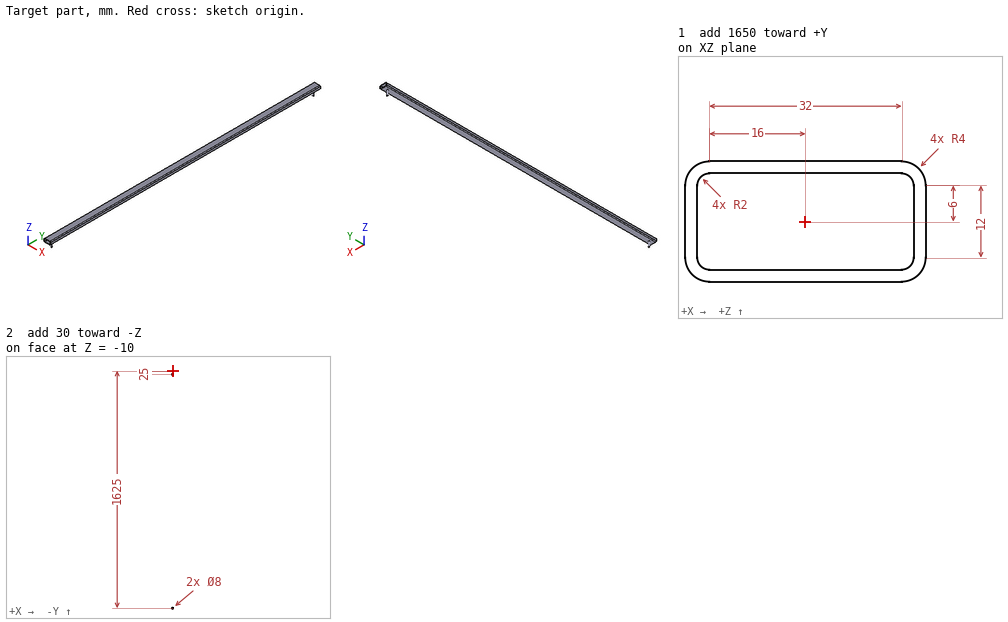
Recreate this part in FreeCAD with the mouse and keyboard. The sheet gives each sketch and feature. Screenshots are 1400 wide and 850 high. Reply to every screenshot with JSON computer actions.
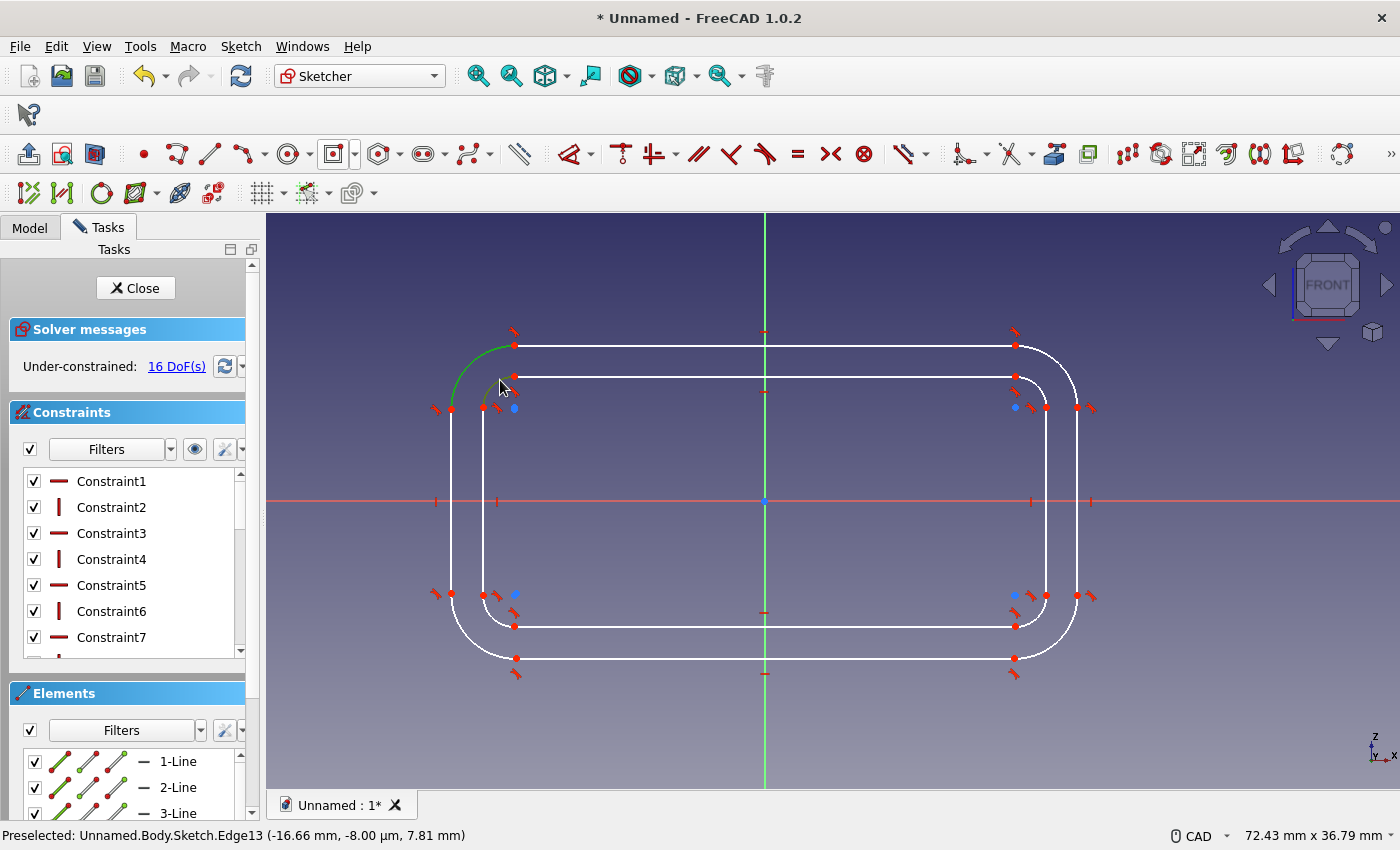
{"action": "left_click", "coordinate": [621, 154]}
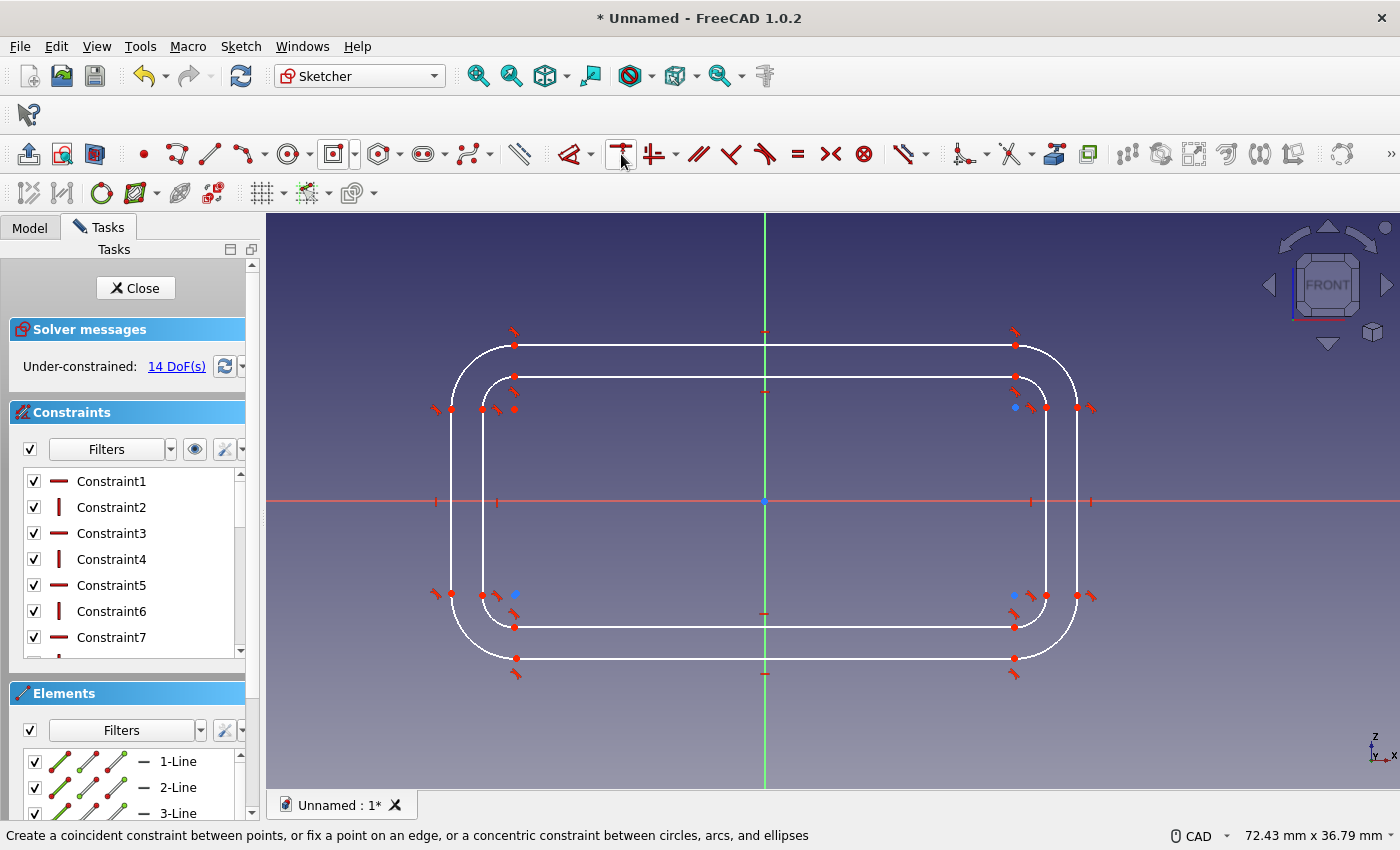
{"action": "left_click", "coordinate": [458, 623]}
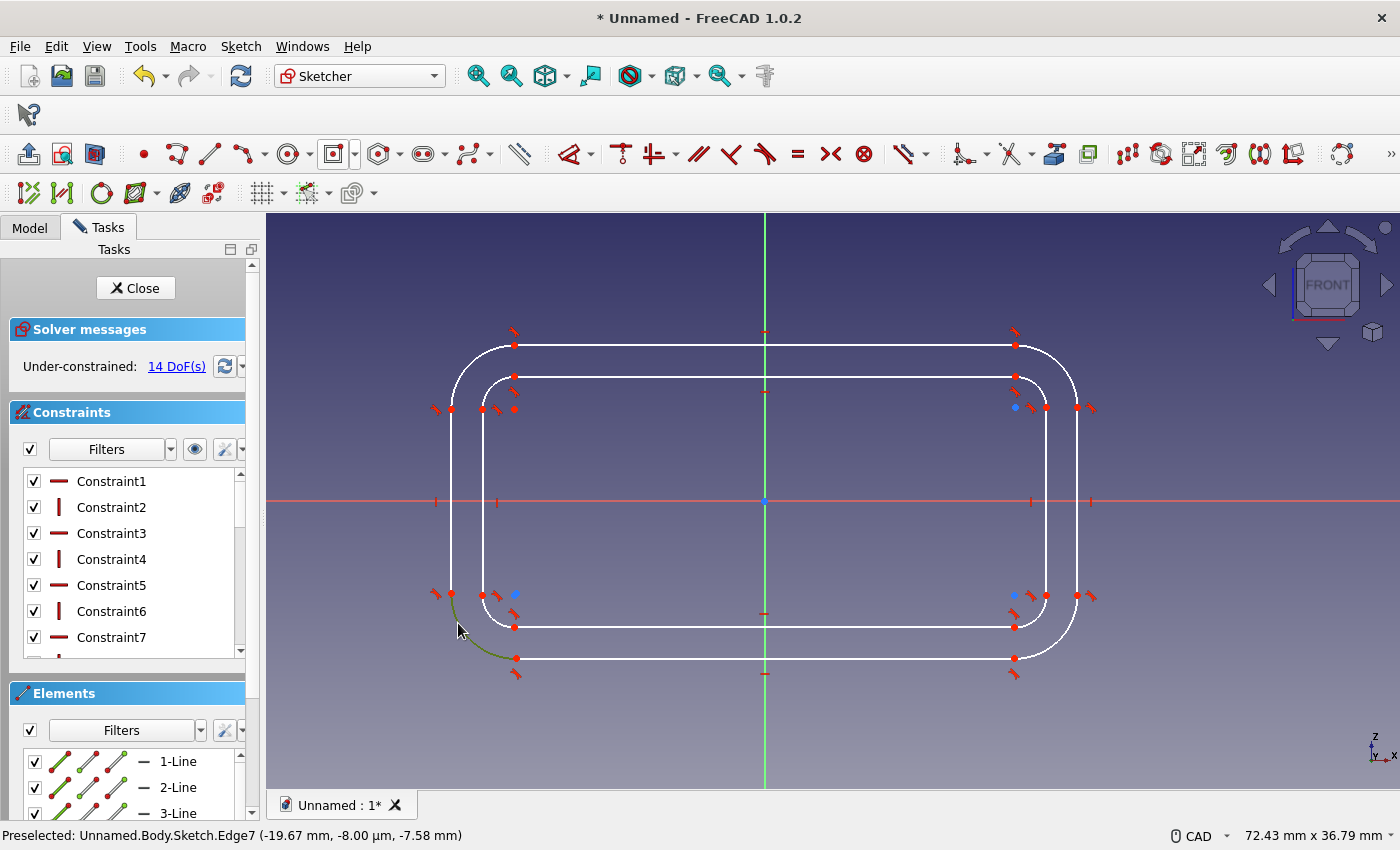
{"action": "left_click", "coordinate": [486, 610]}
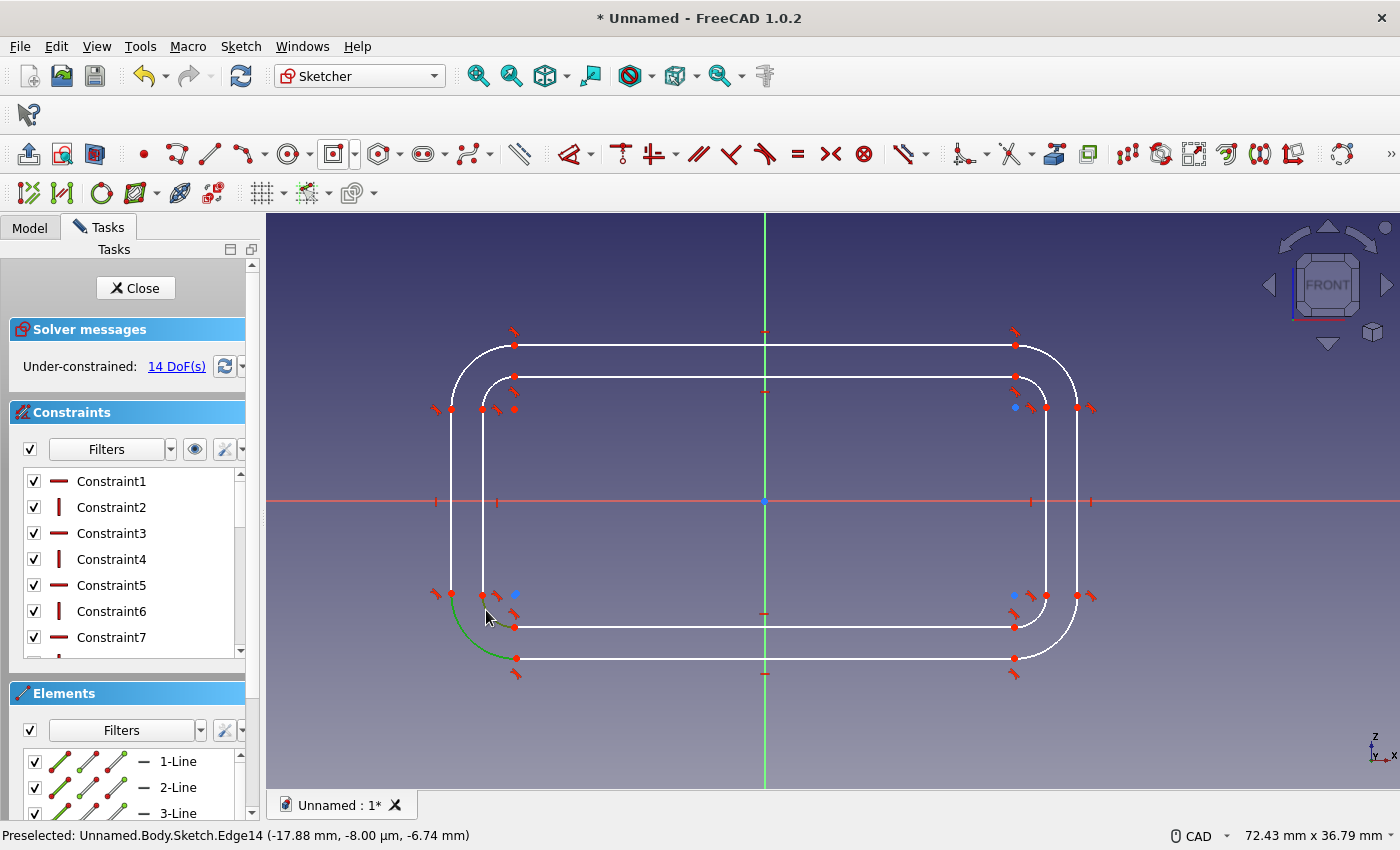
{"action": "key", "text": "c"}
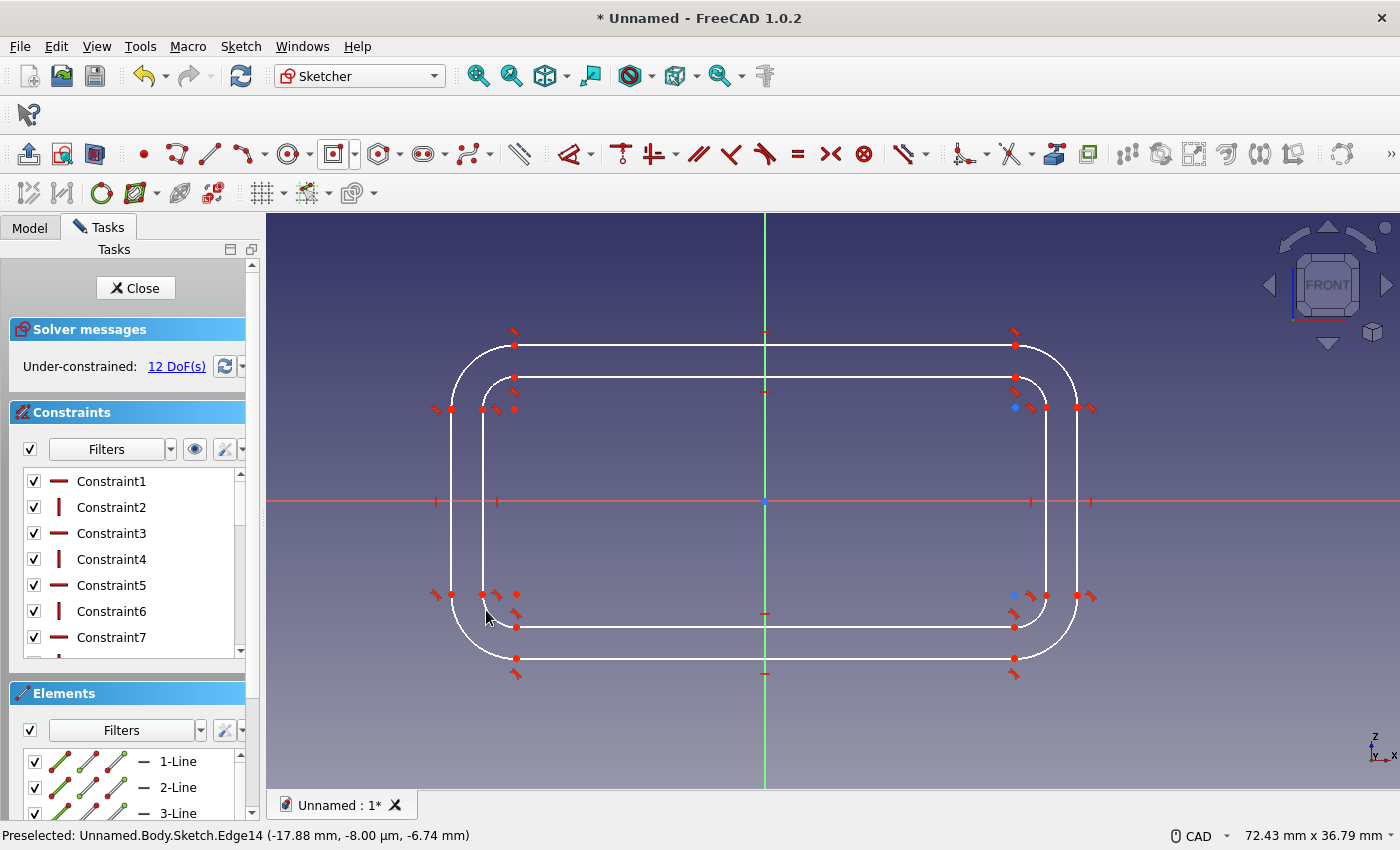
{"action": "left_click", "coordinate": [1043, 652]}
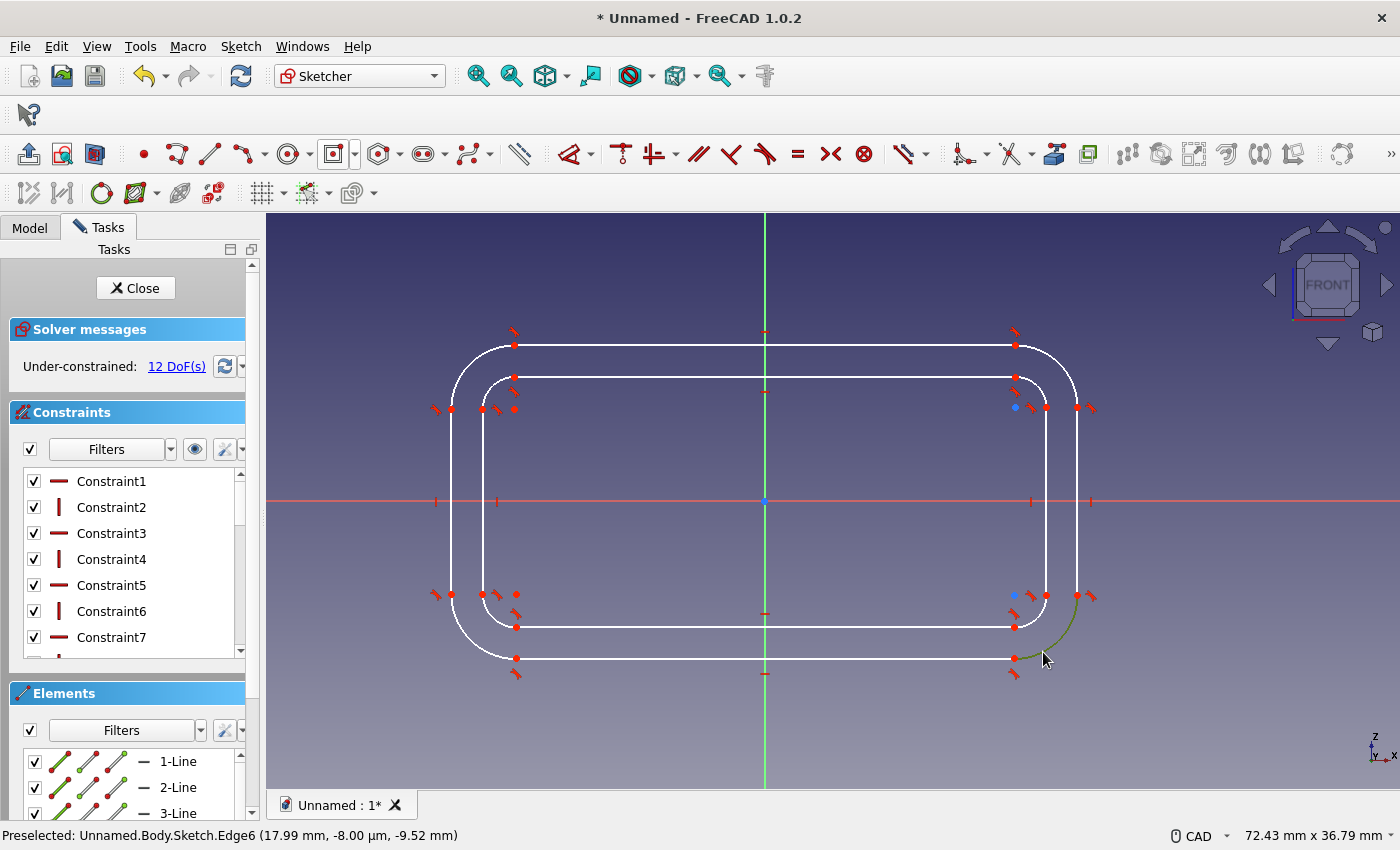
{"action": "left_click", "coordinate": [1029, 624]}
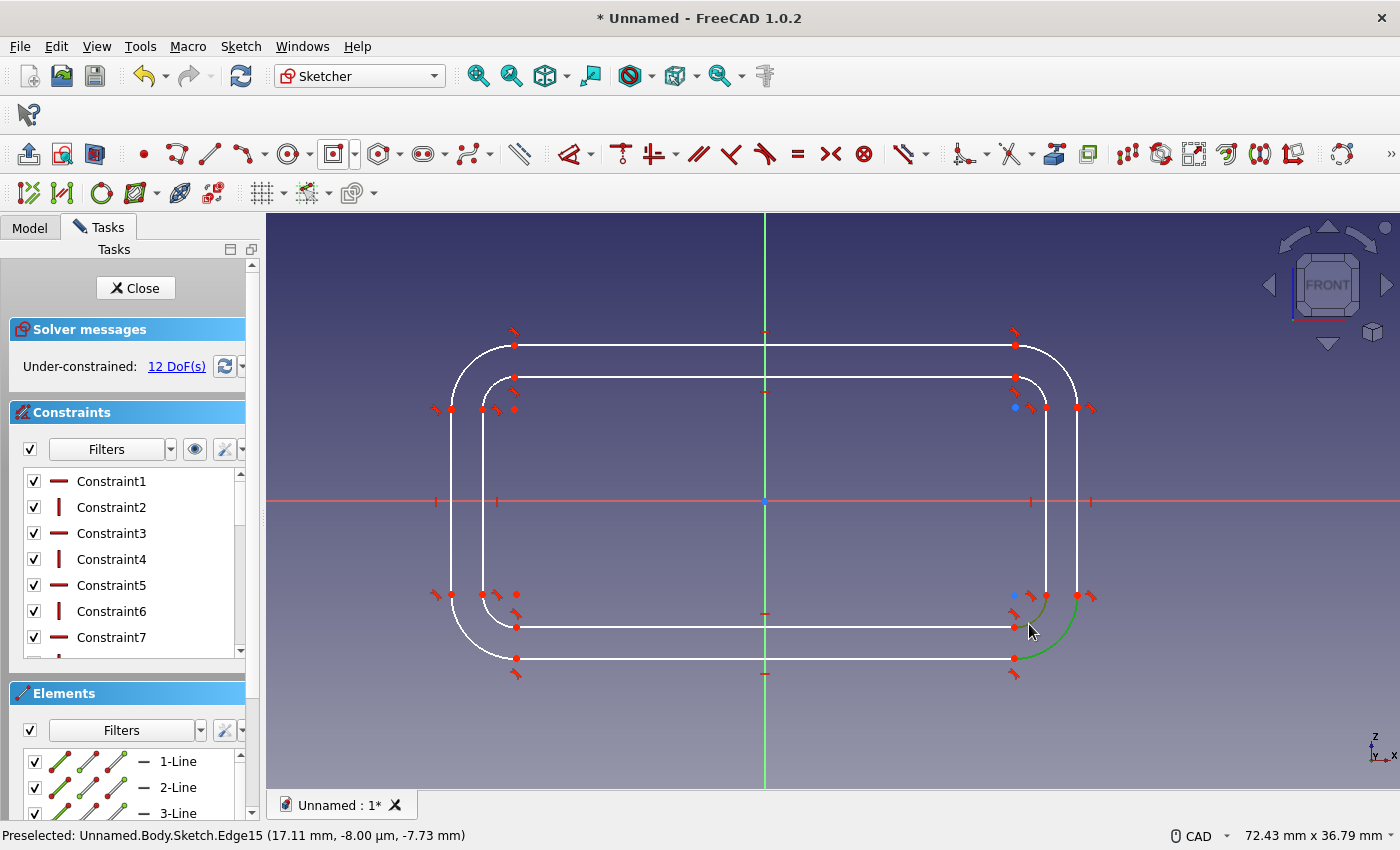
{"action": "left_click", "coordinate": [621, 154]}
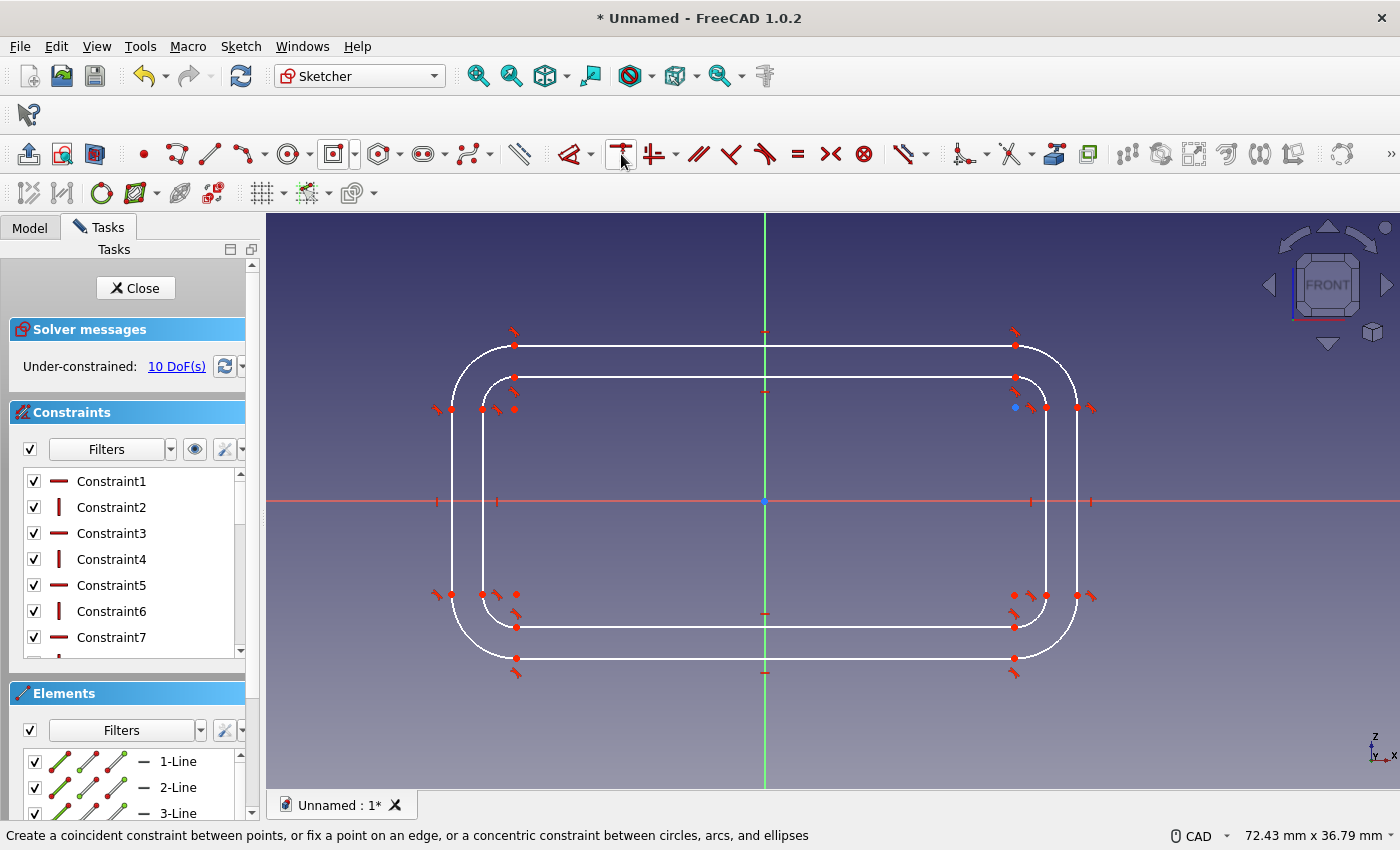
{"action": "left_click", "coordinate": [1071, 380]}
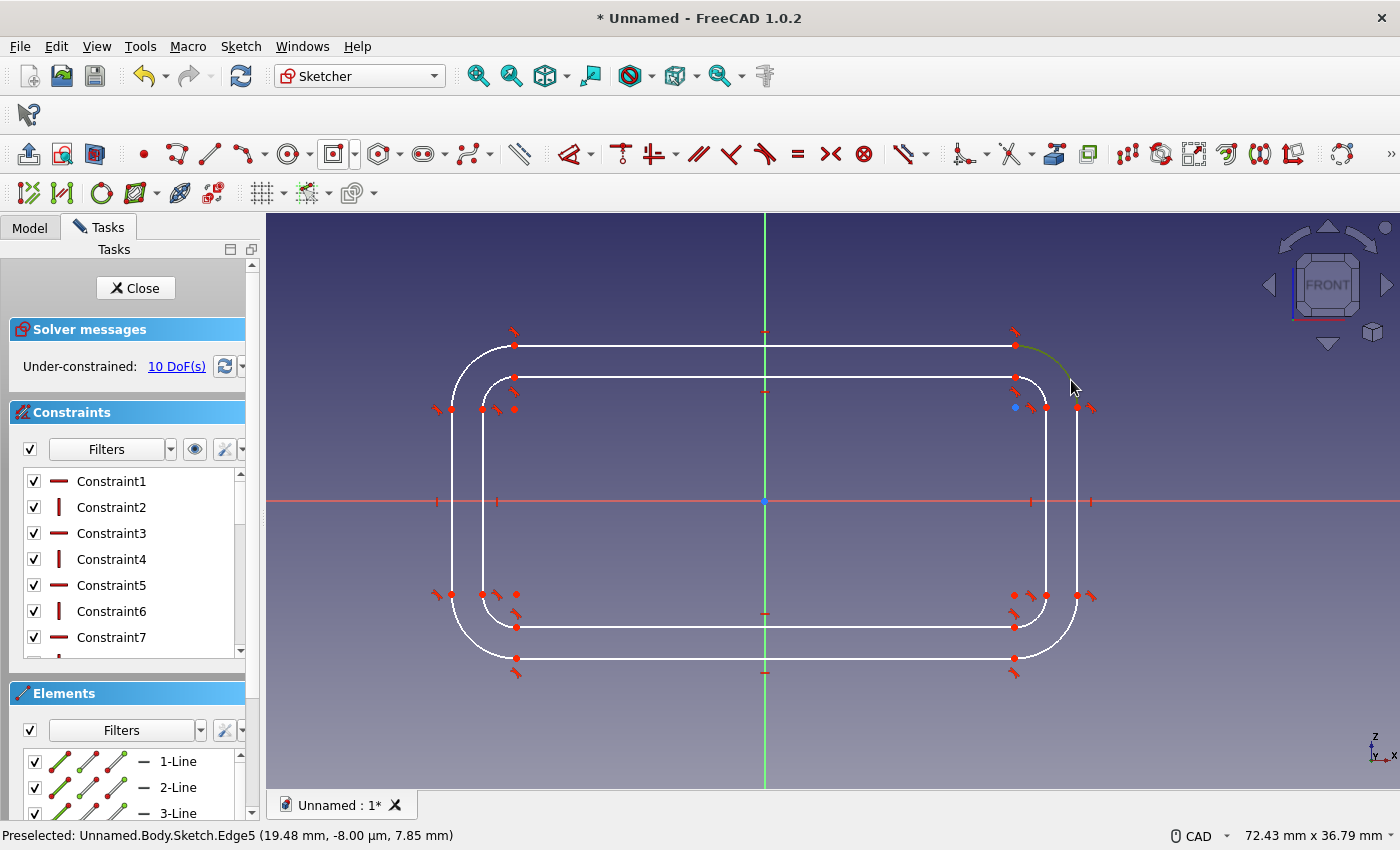
{"action": "left_click", "coordinate": [1043, 652]}